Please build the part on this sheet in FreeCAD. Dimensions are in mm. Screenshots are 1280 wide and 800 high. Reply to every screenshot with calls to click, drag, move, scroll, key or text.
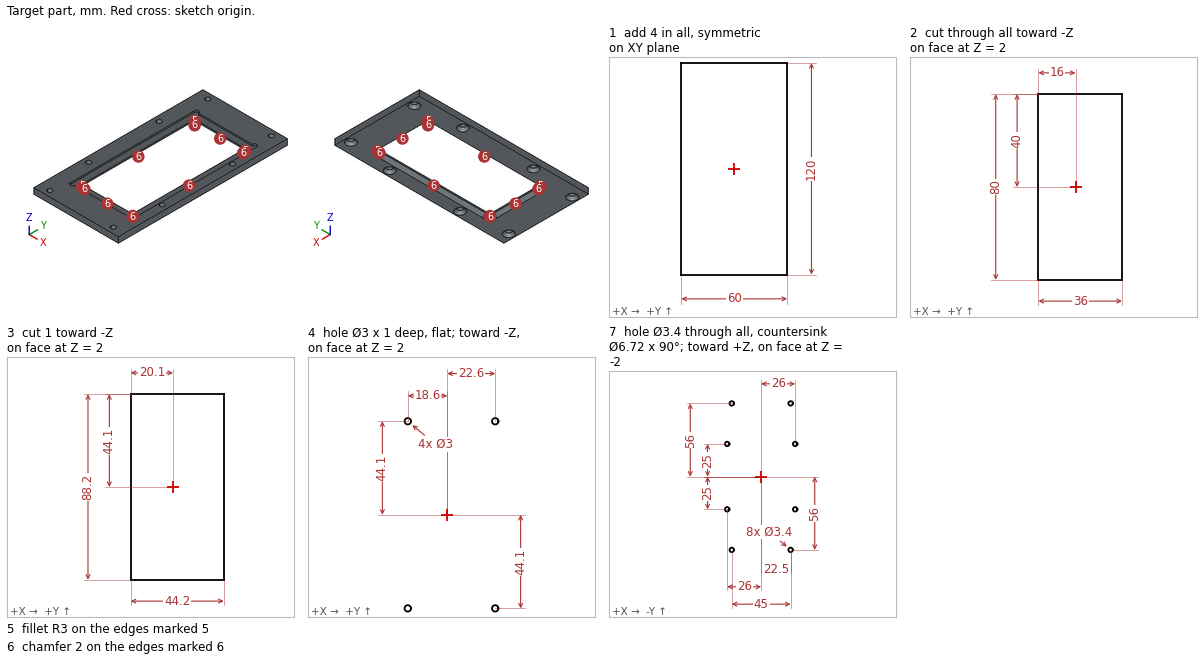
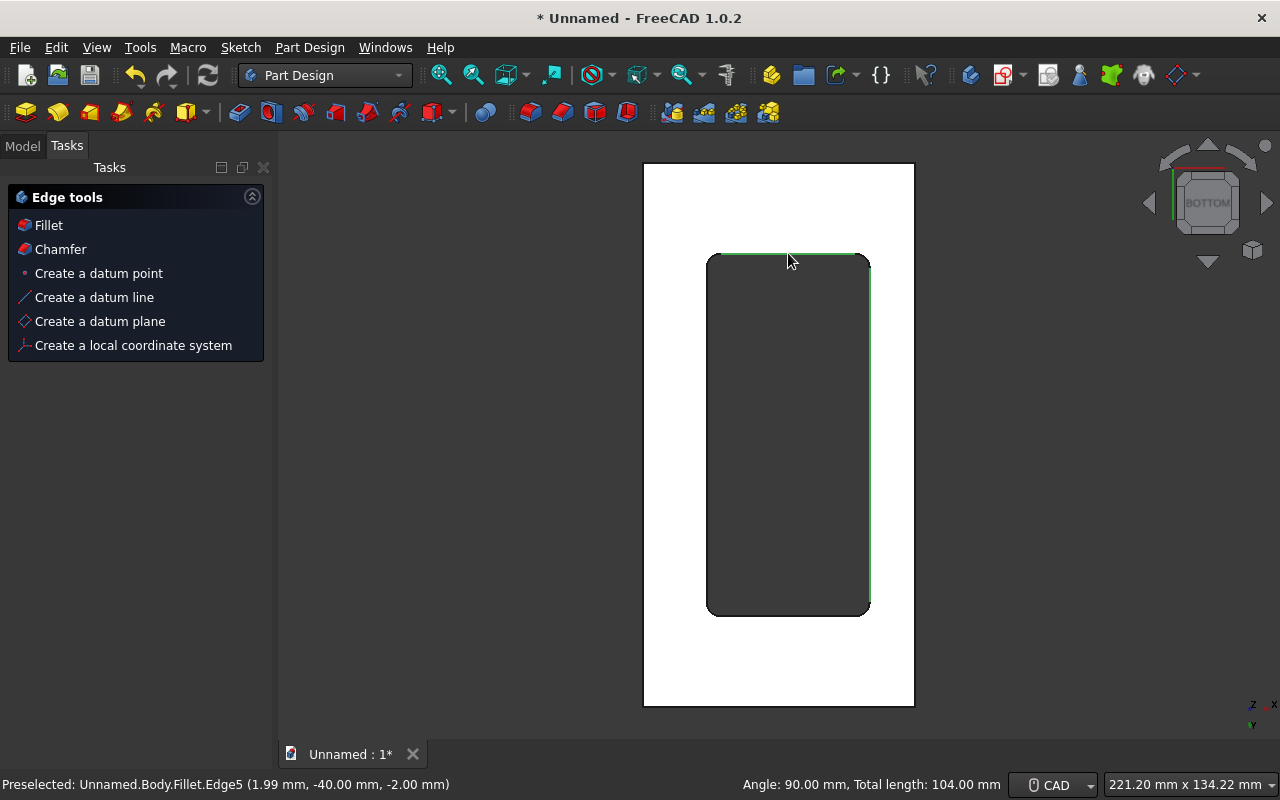
click(707, 434, ctrl)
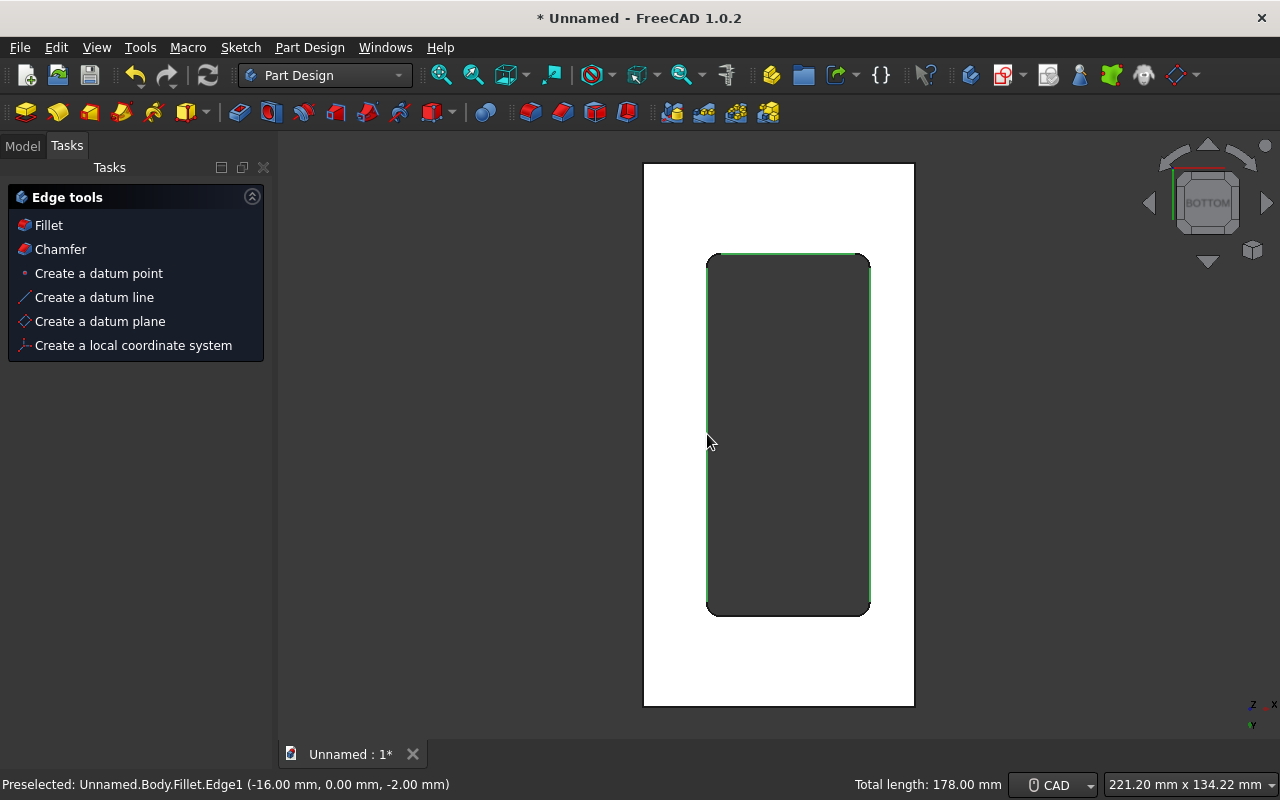
click(866, 611, ctrl)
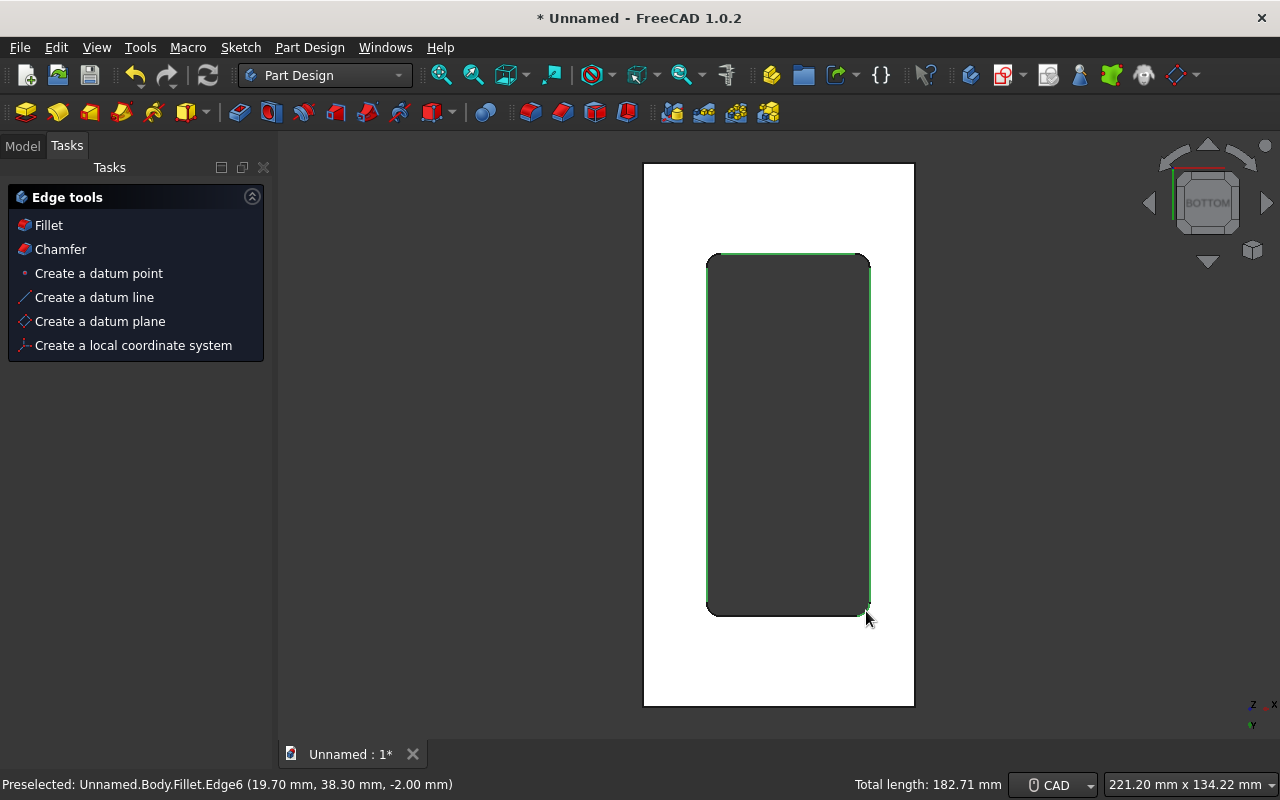
click(866, 257, ctrl)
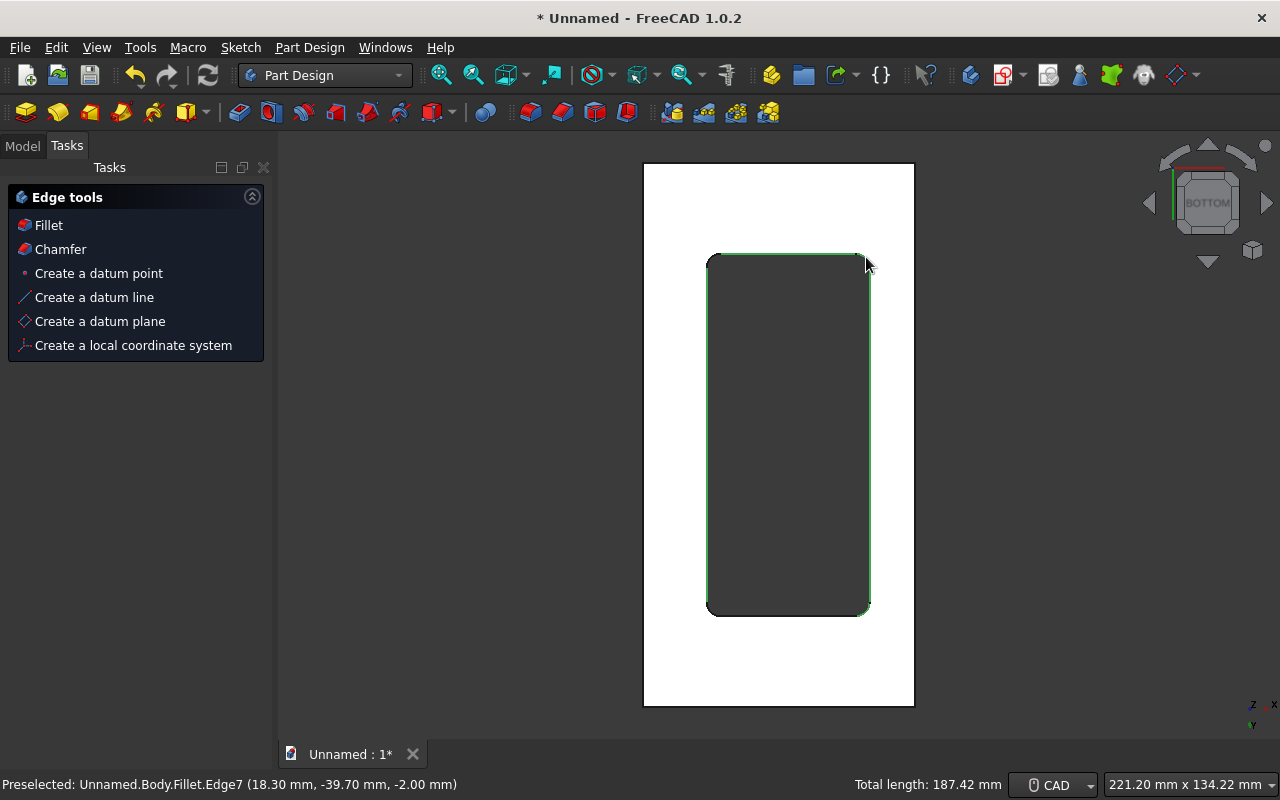
click(711, 257, ctrl)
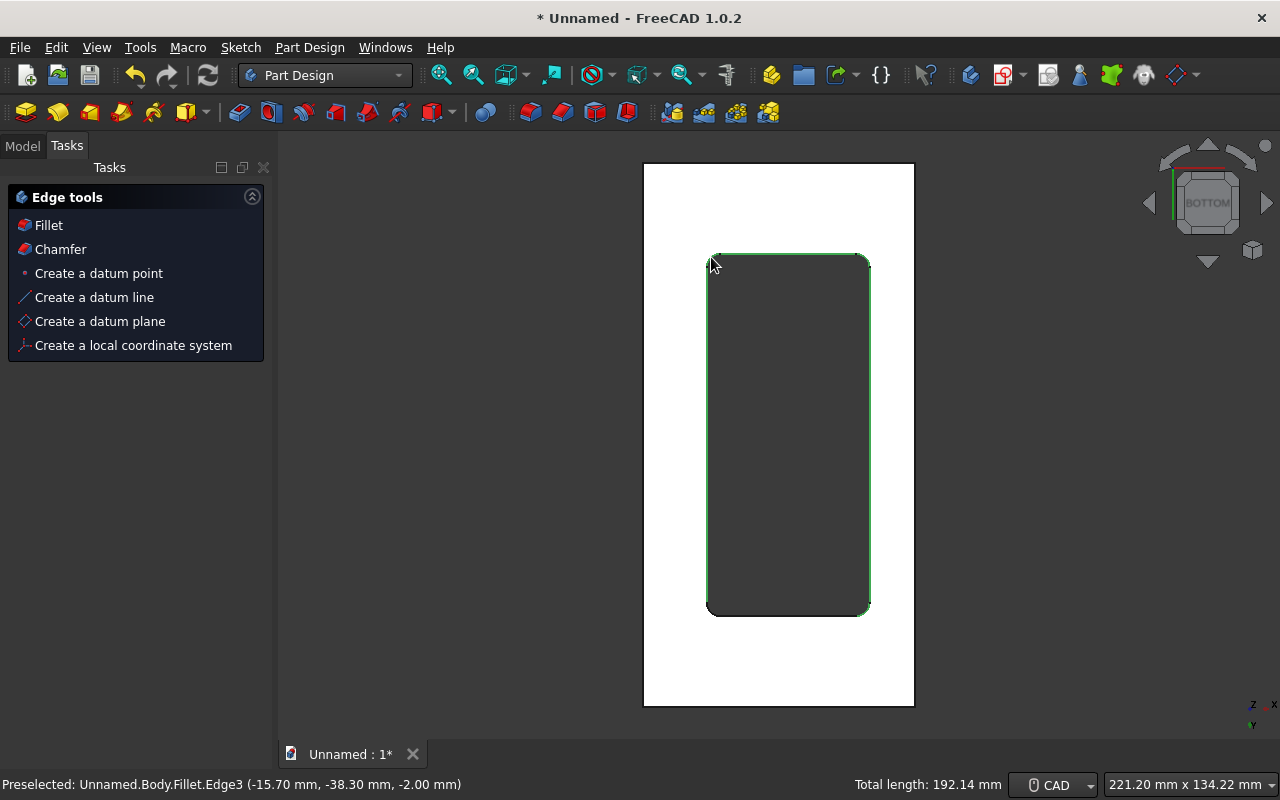
click(711, 611, ctrl)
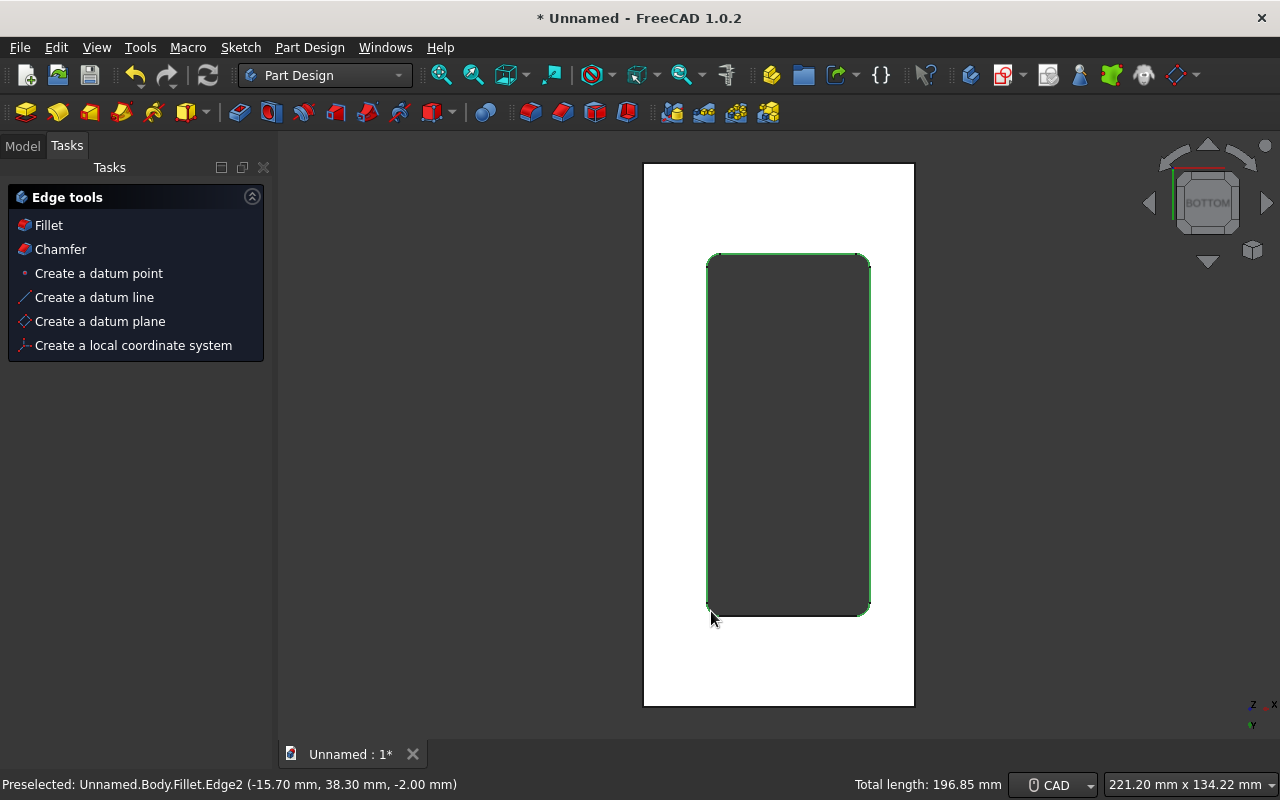
click(788, 615, ctrl)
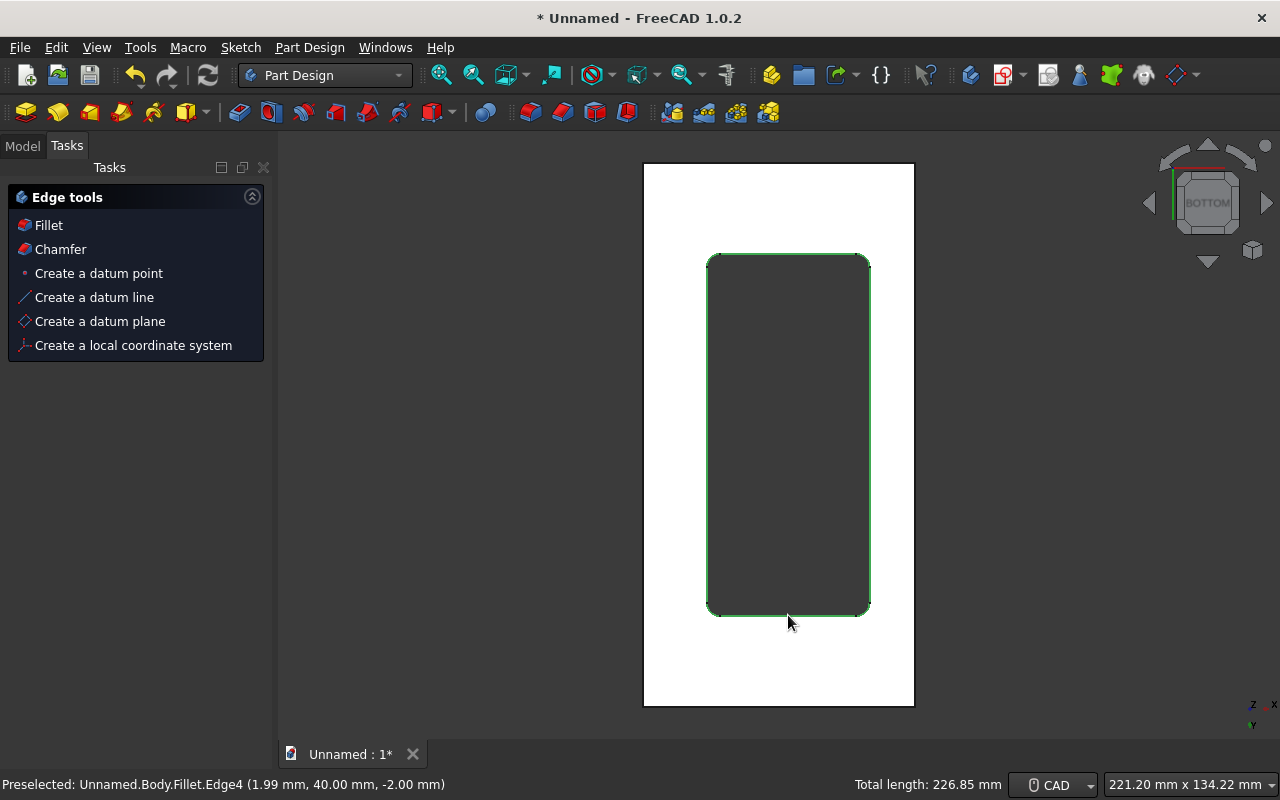
click(564, 112)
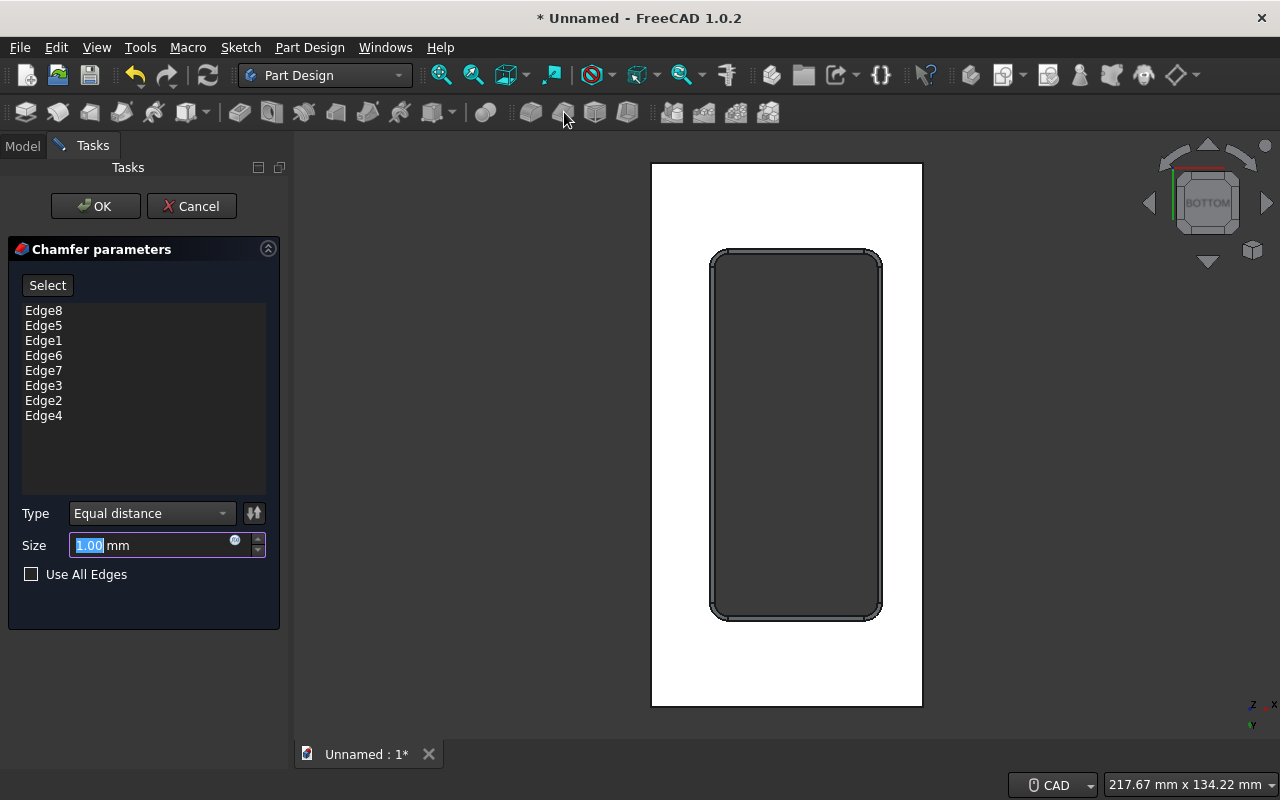
text(2)
key(Tab)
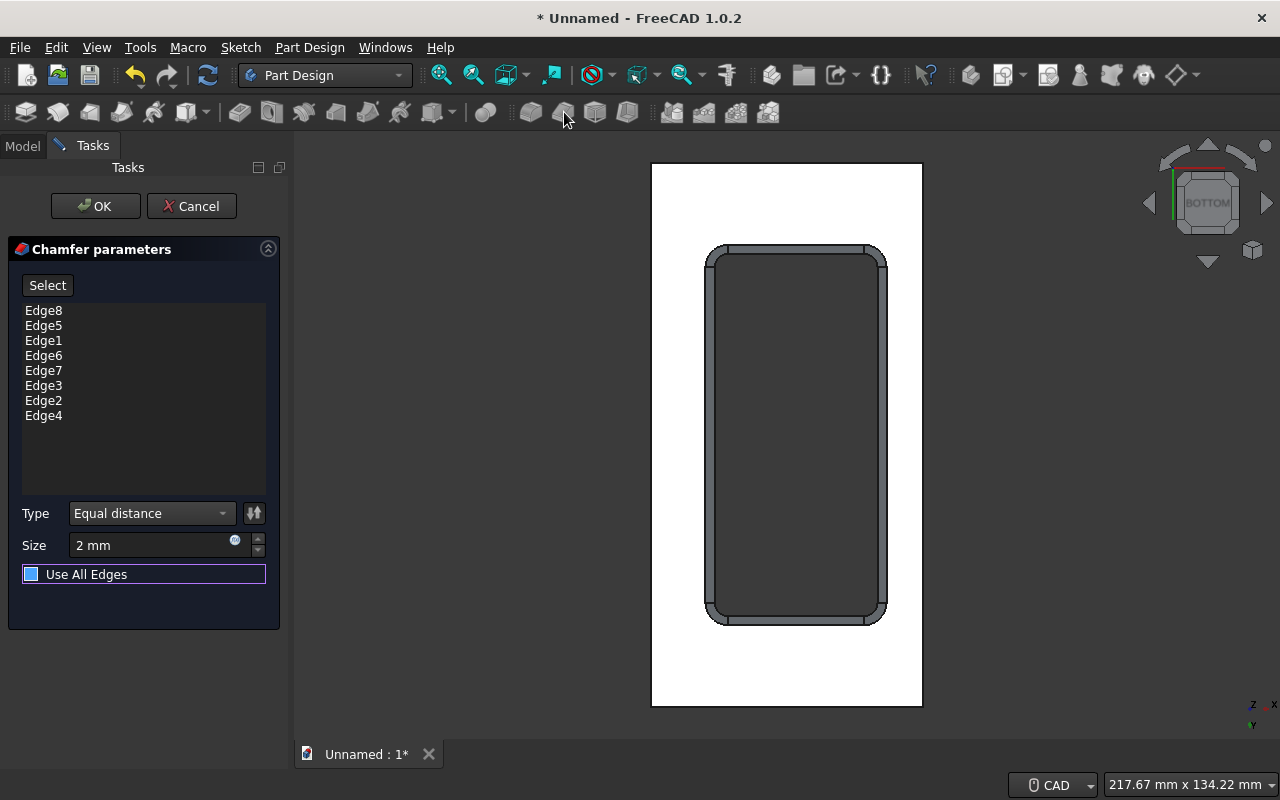
click(96, 206)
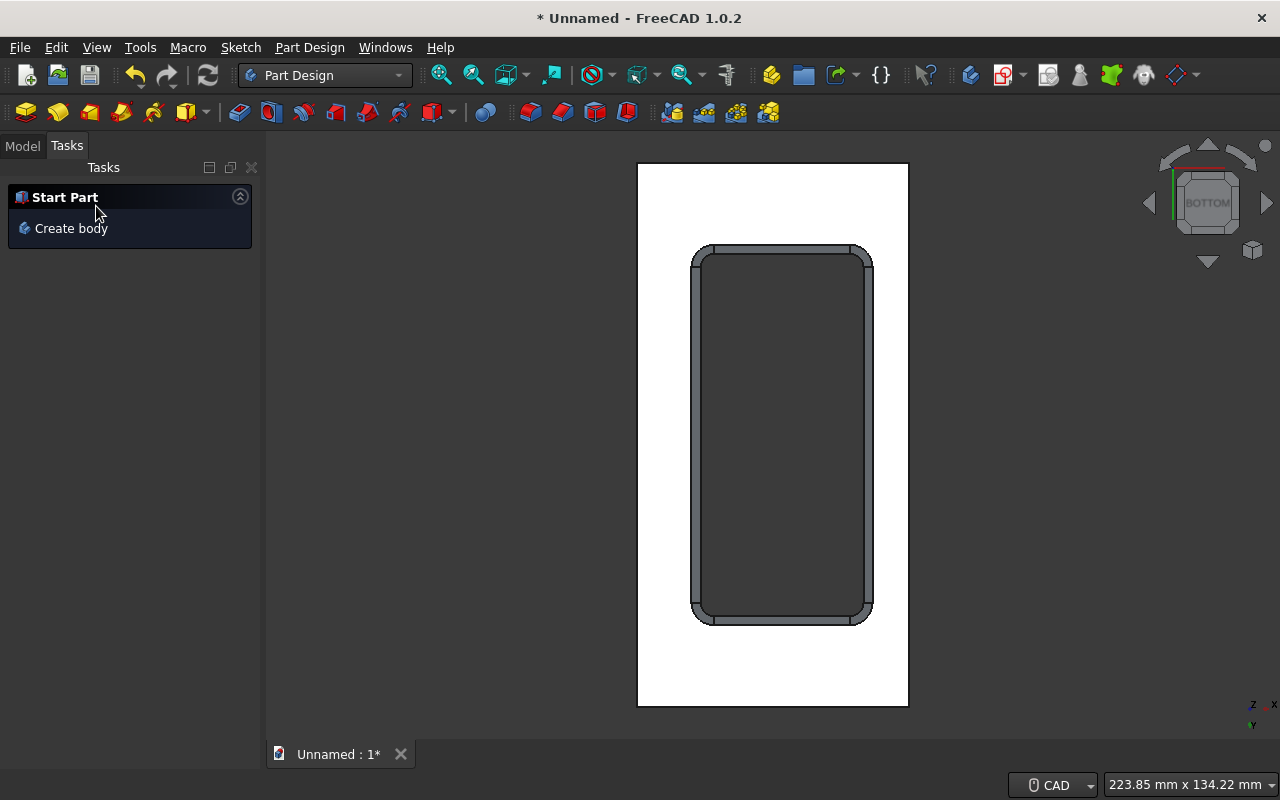
click(851, 667)